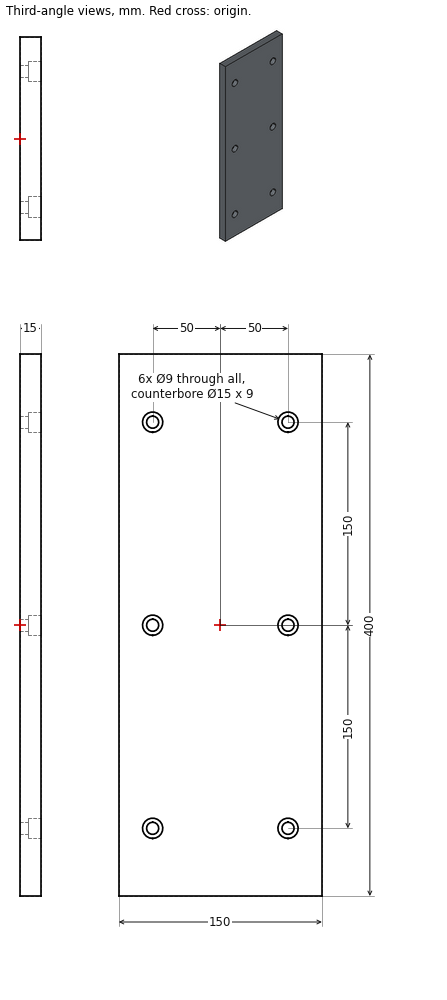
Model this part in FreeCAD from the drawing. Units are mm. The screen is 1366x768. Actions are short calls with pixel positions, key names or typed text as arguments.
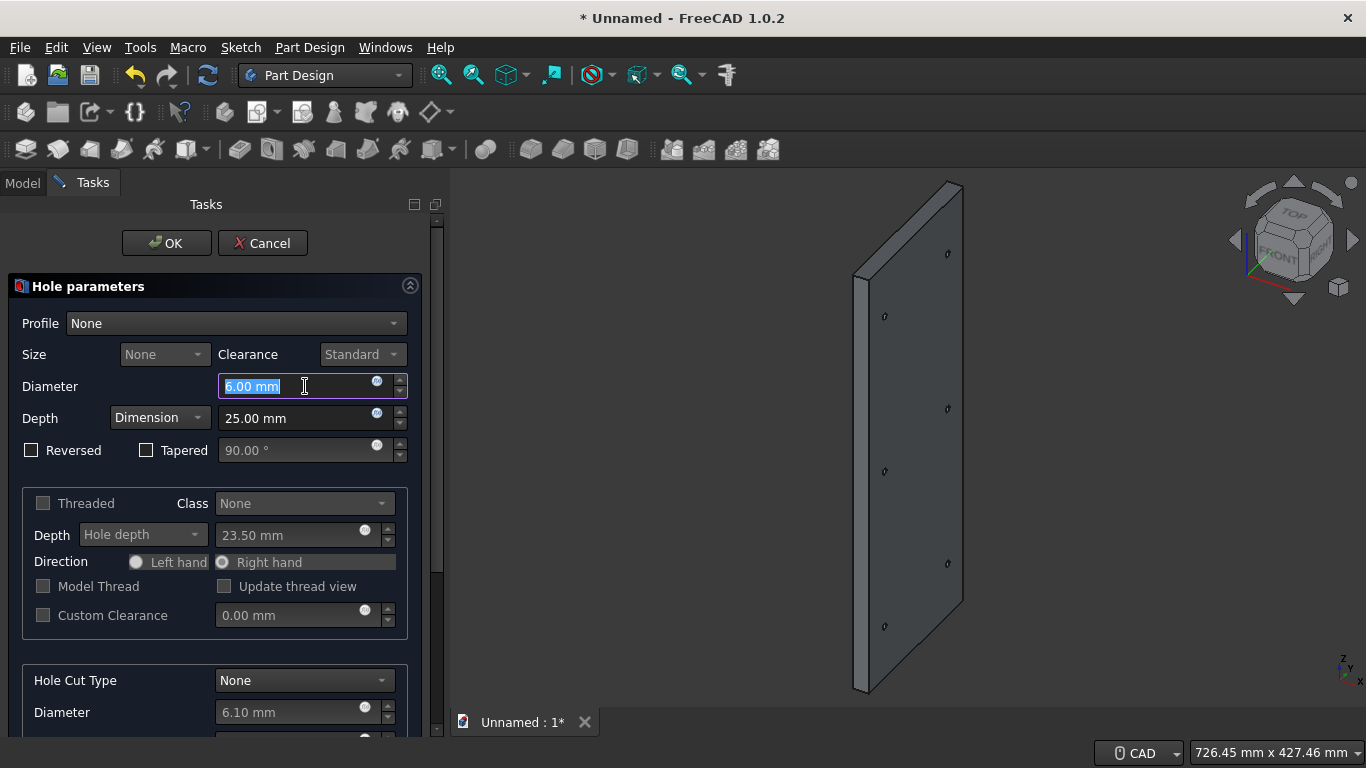
text(9)
key(Tab)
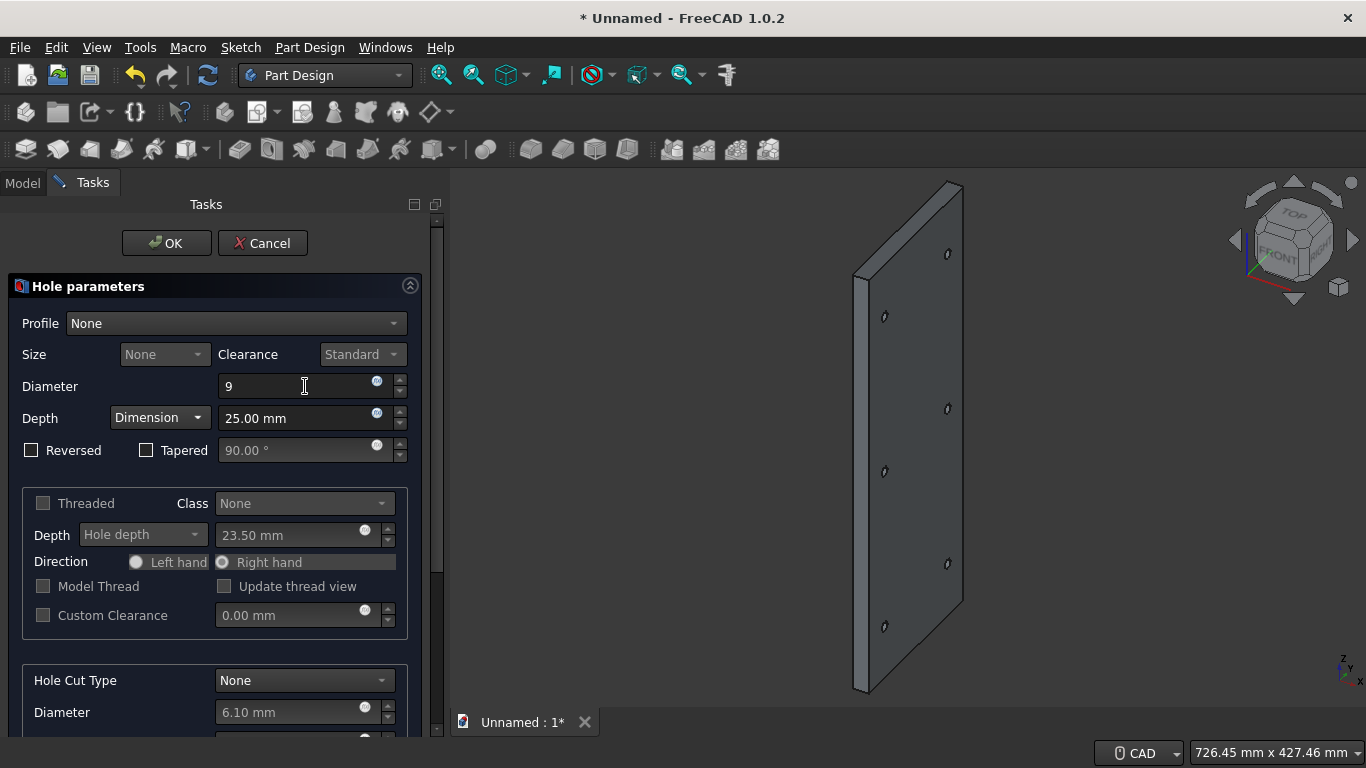
click(161, 418)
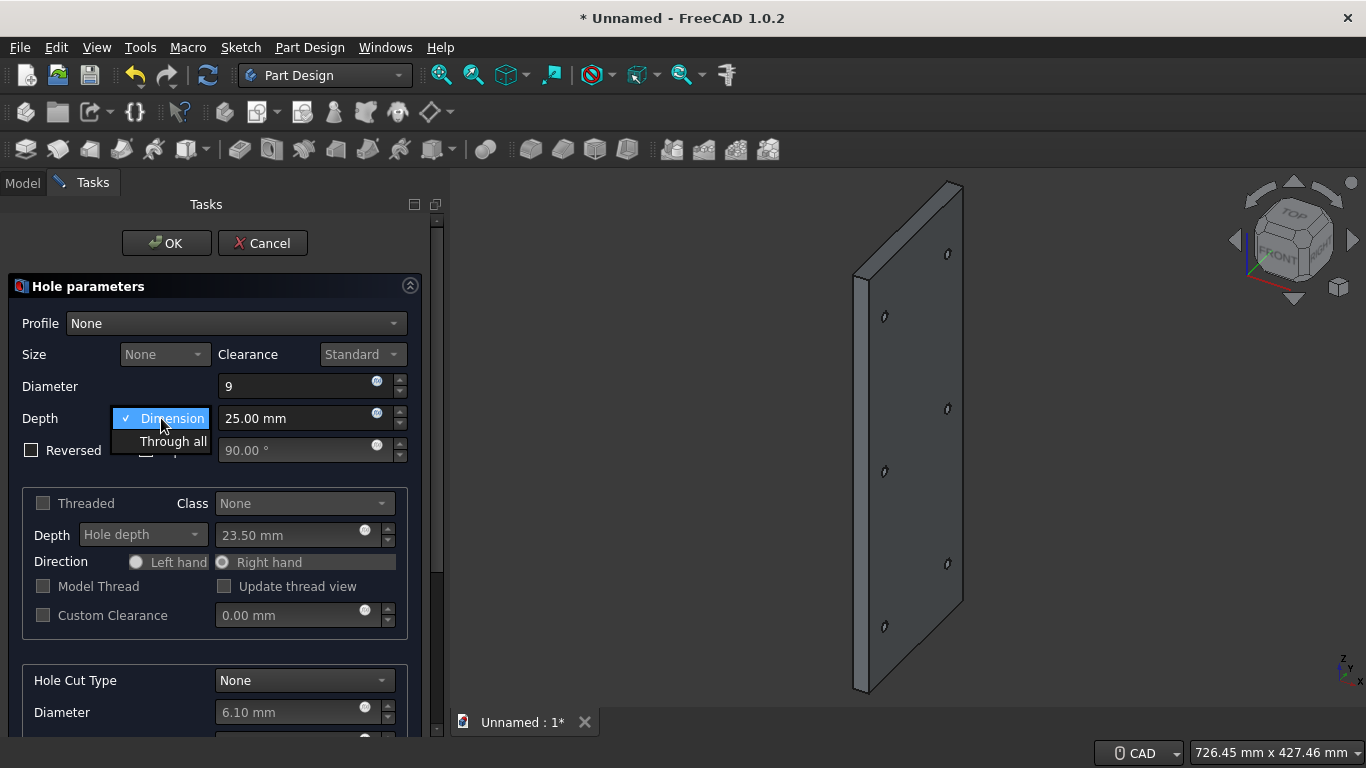
click(160, 442)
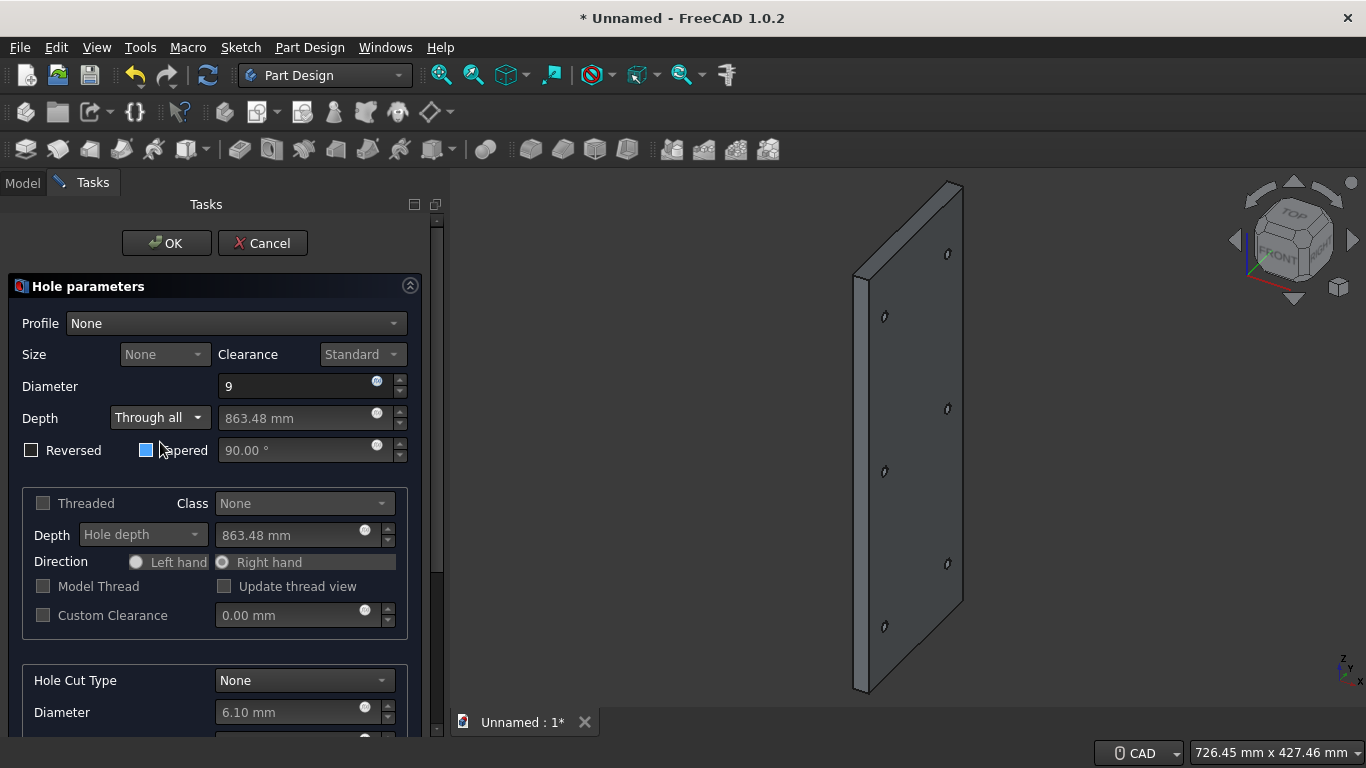
click(306, 680)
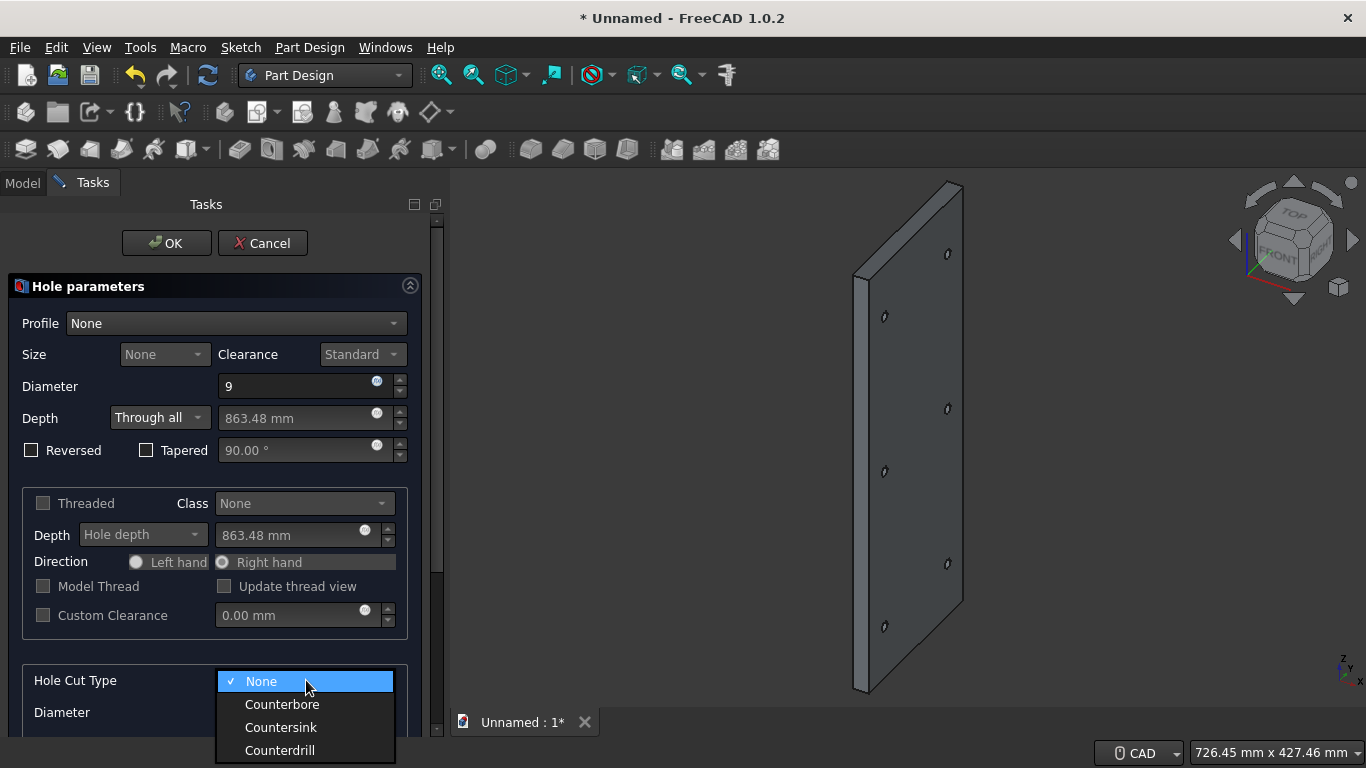
click(304, 704)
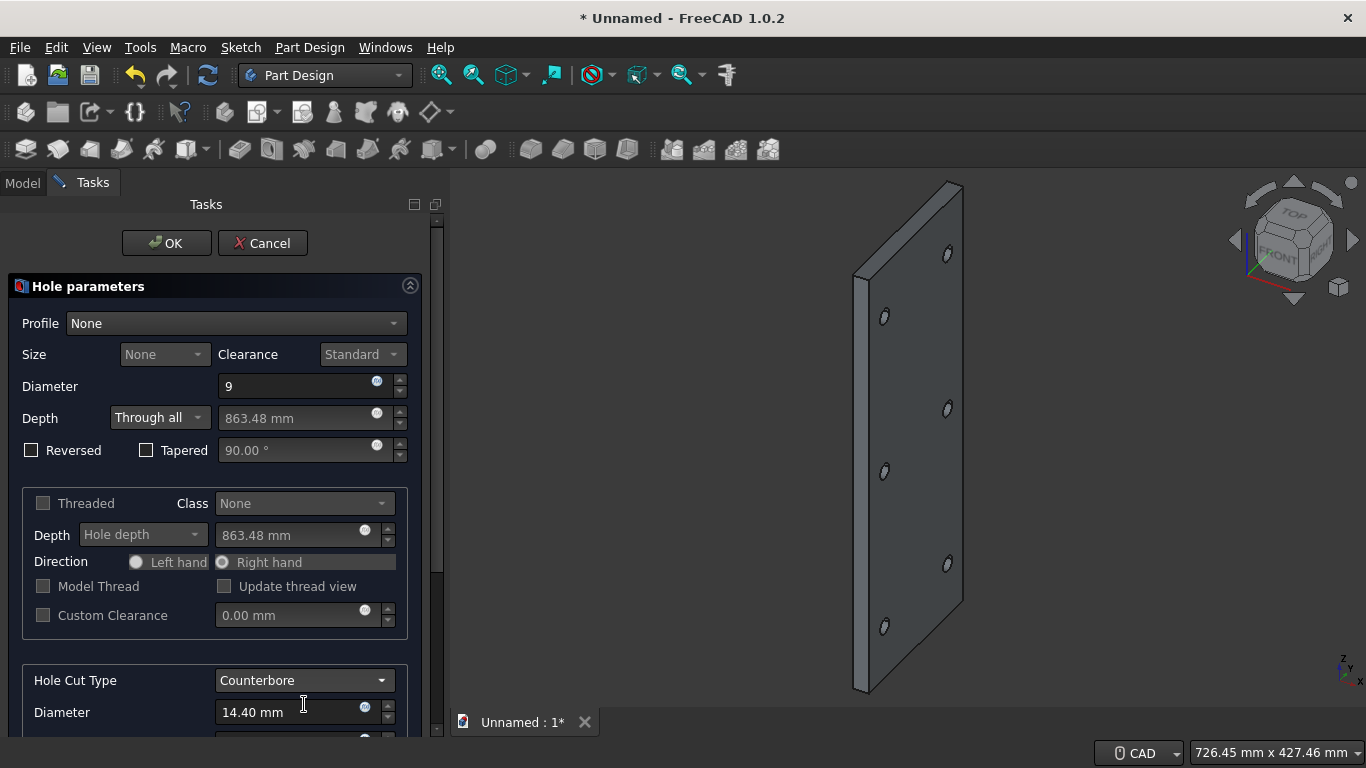
triple_click(298, 712)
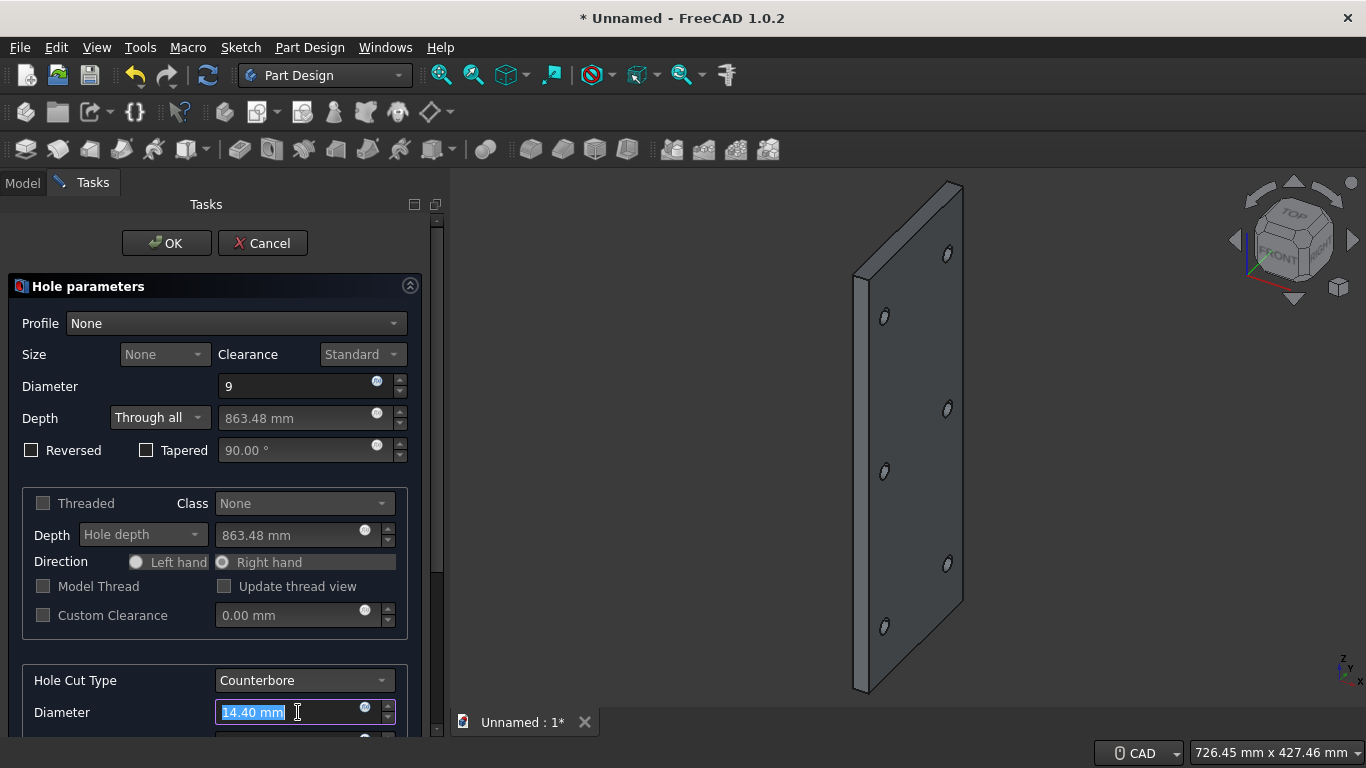
text(15)
key(Tab)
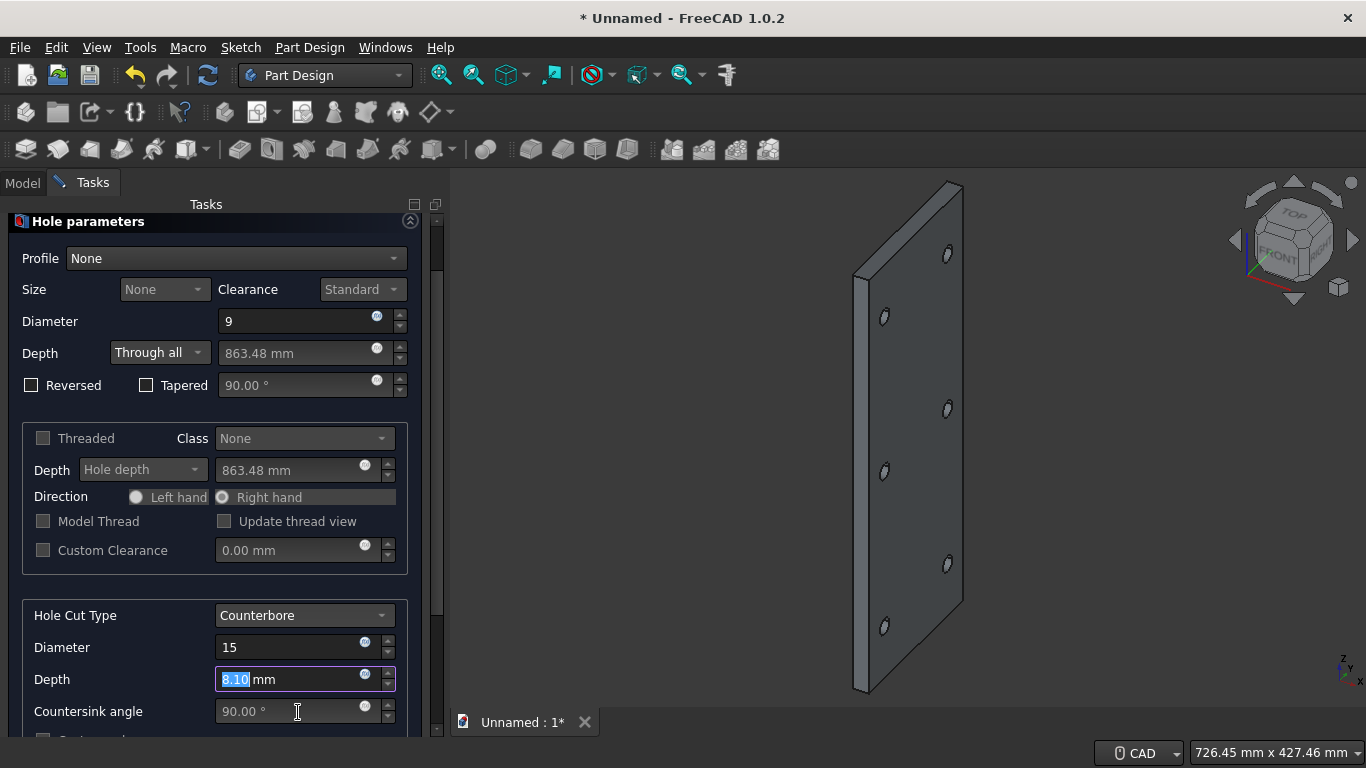
text(9)
key(Tab)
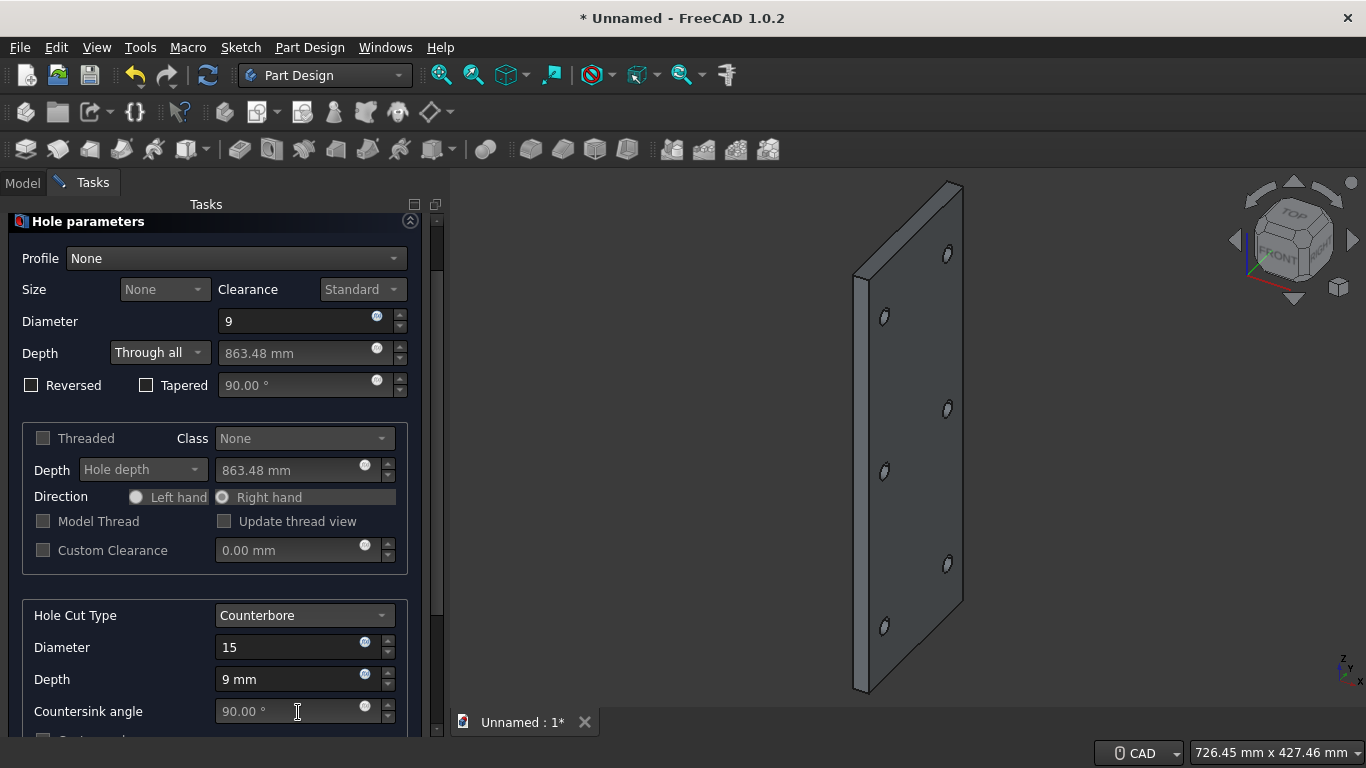
scroll(437, 475, up, 2)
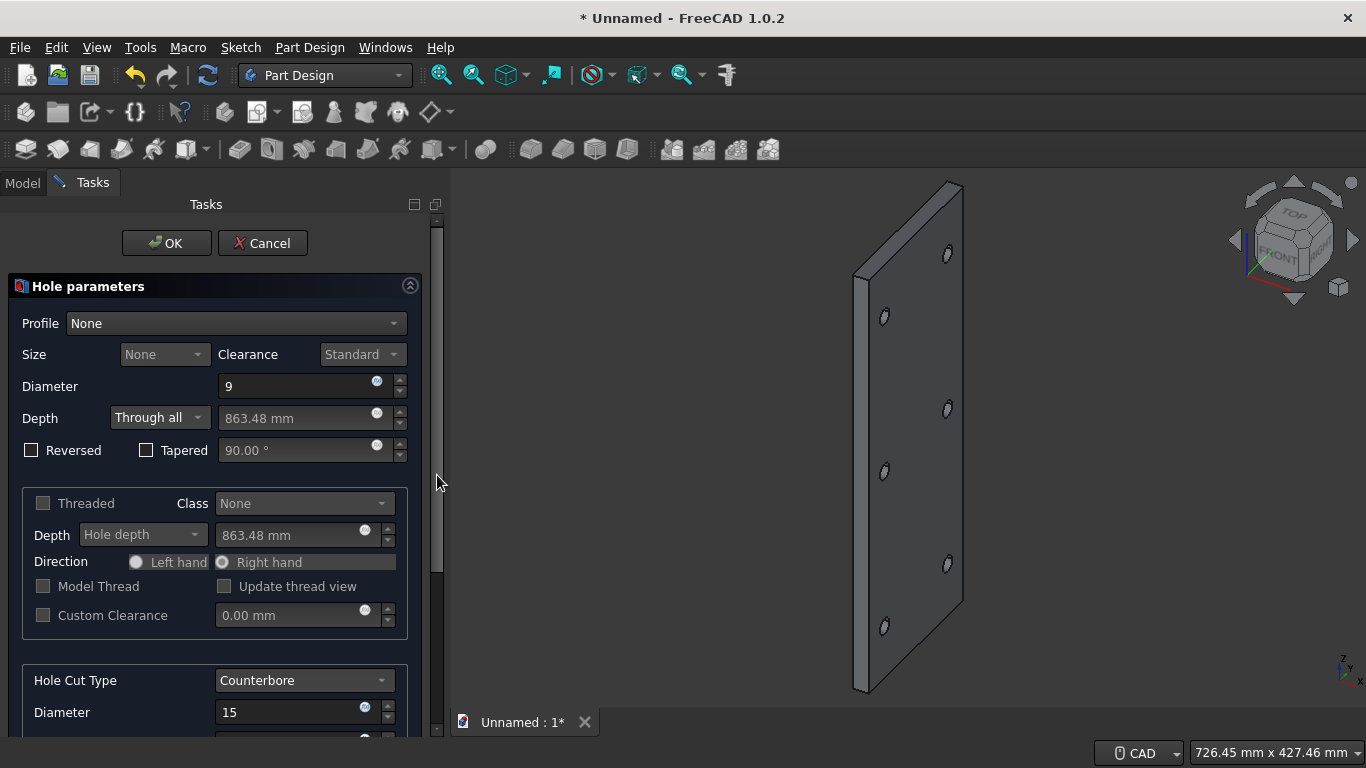
click(167, 243)